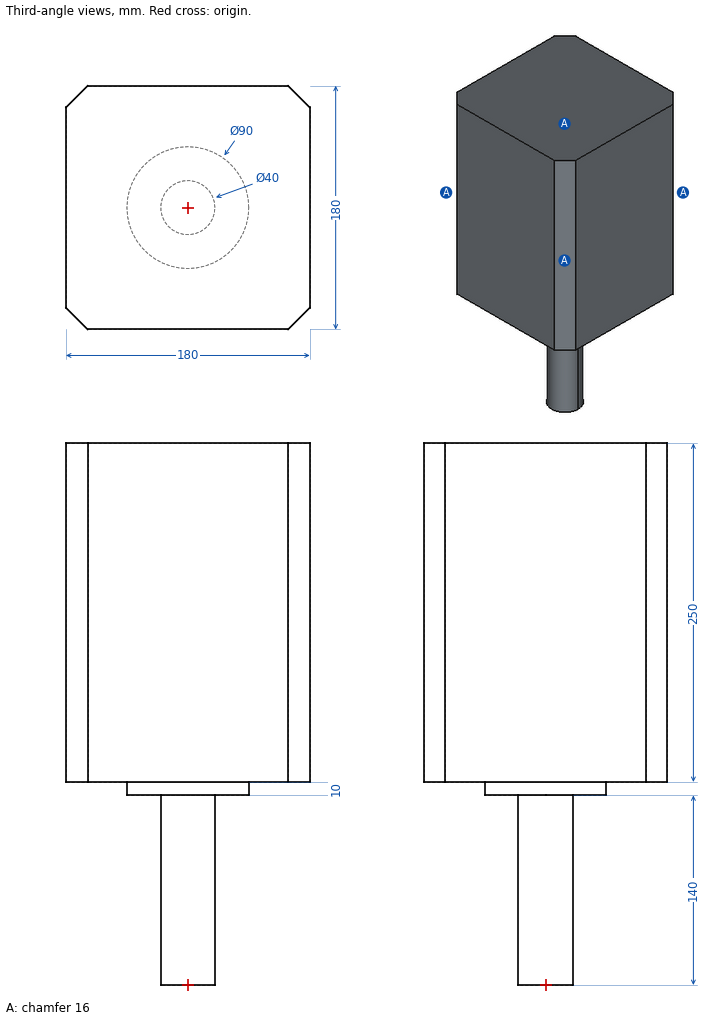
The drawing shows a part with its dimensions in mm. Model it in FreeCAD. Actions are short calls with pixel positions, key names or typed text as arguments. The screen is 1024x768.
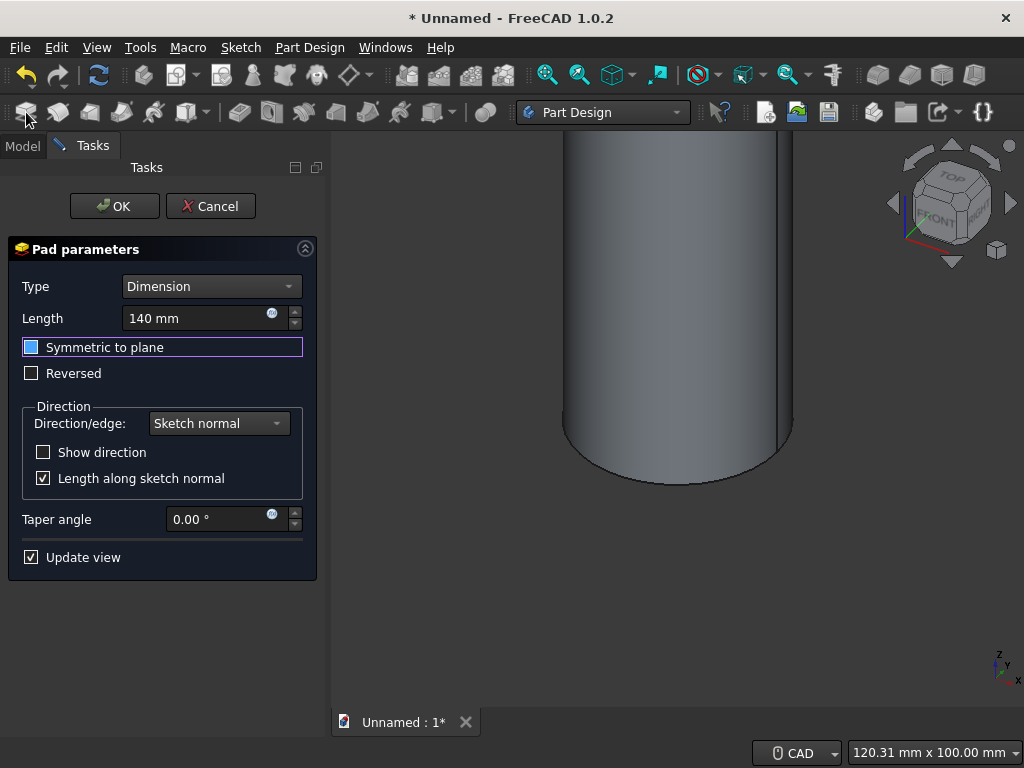
click(115, 206)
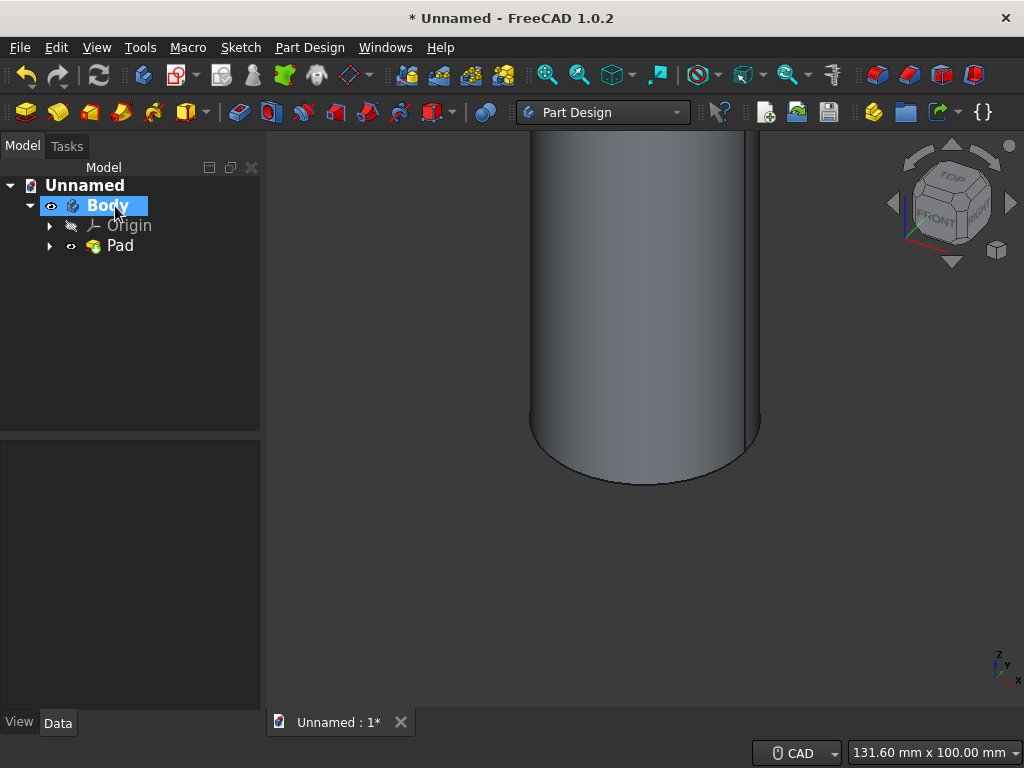
click(548, 76)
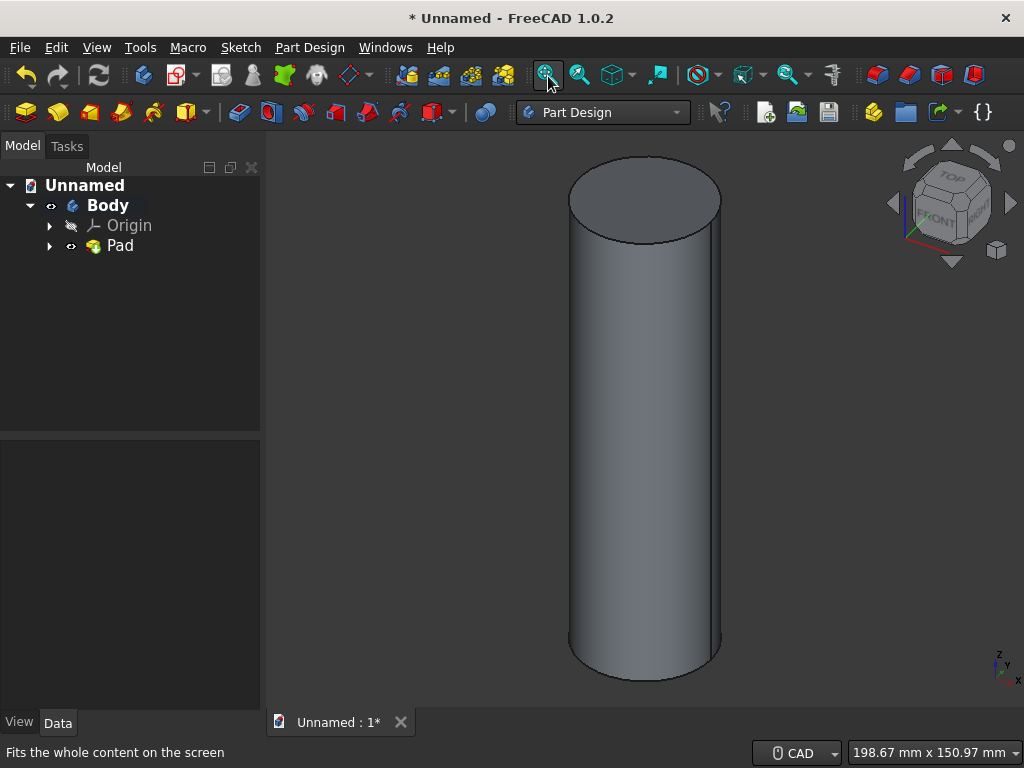
click(645, 199)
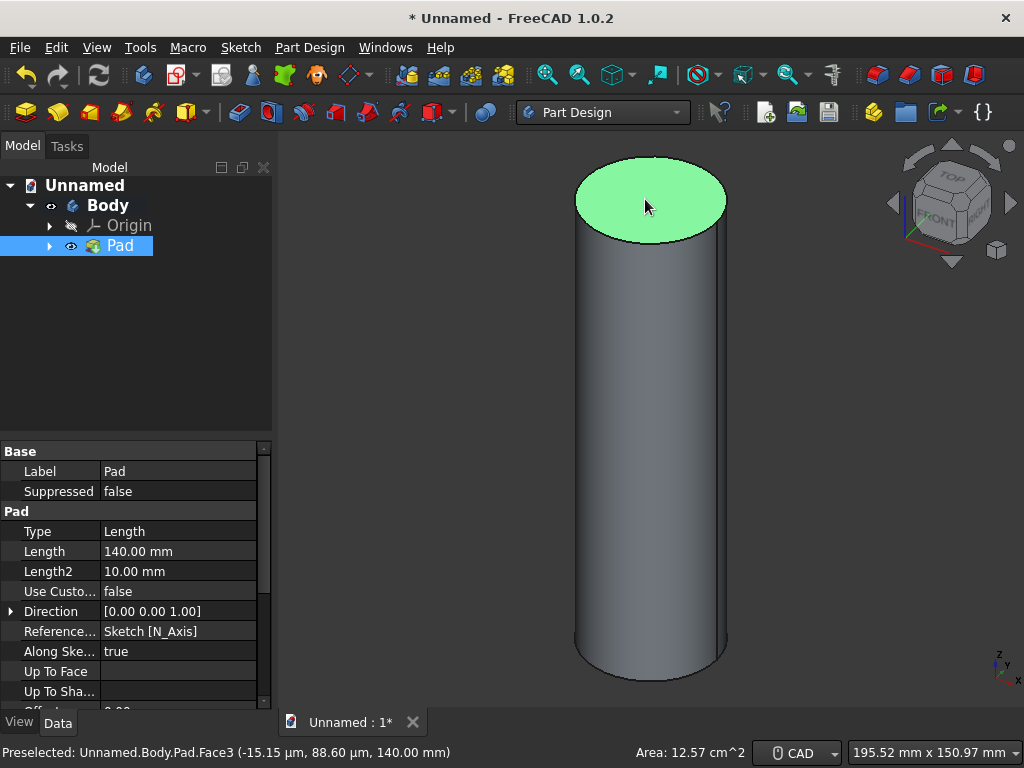
click(176, 76)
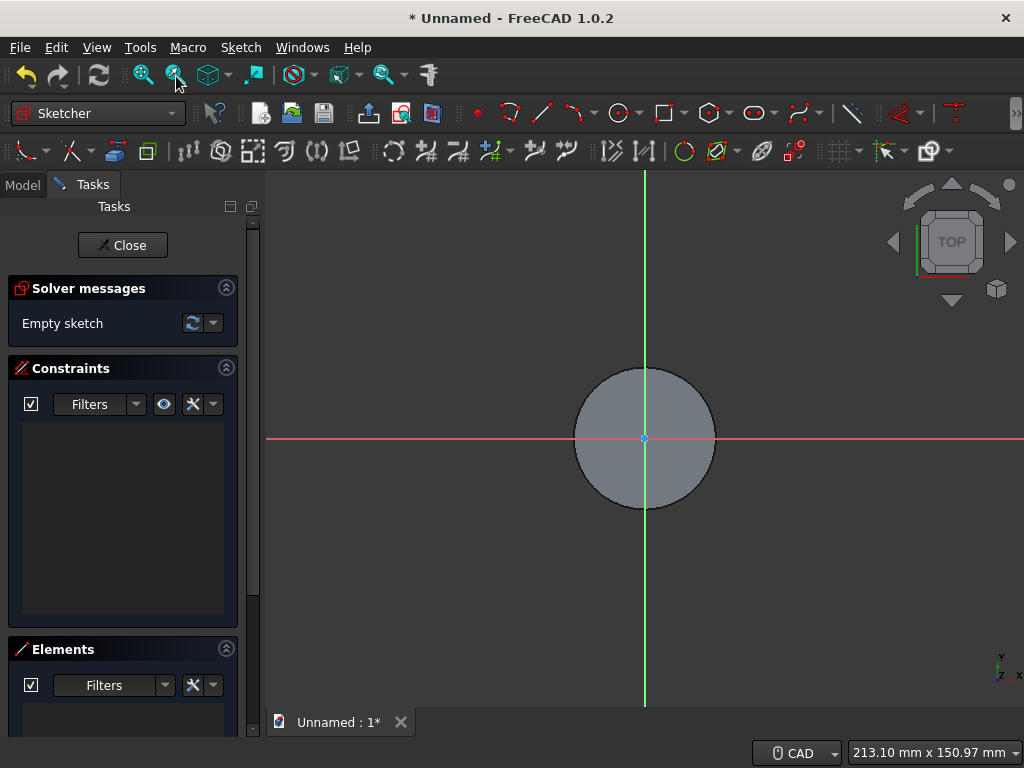
click(620, 114)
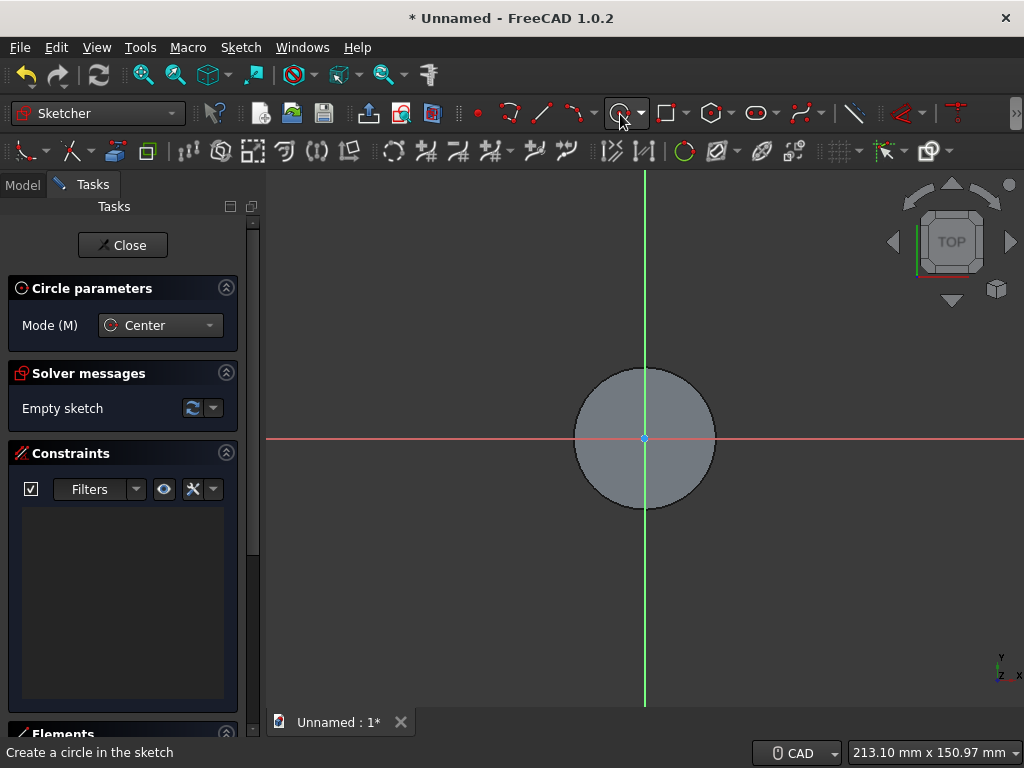
click(645, 438)
click(758, 325)
key(Escape)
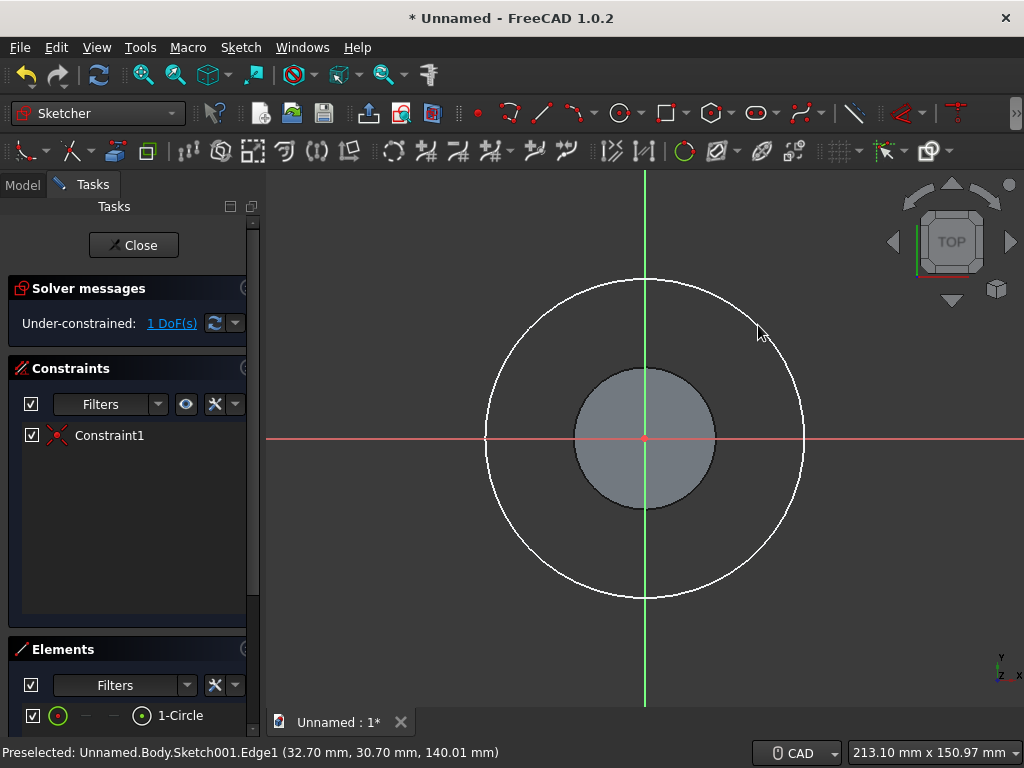
click(902, 114)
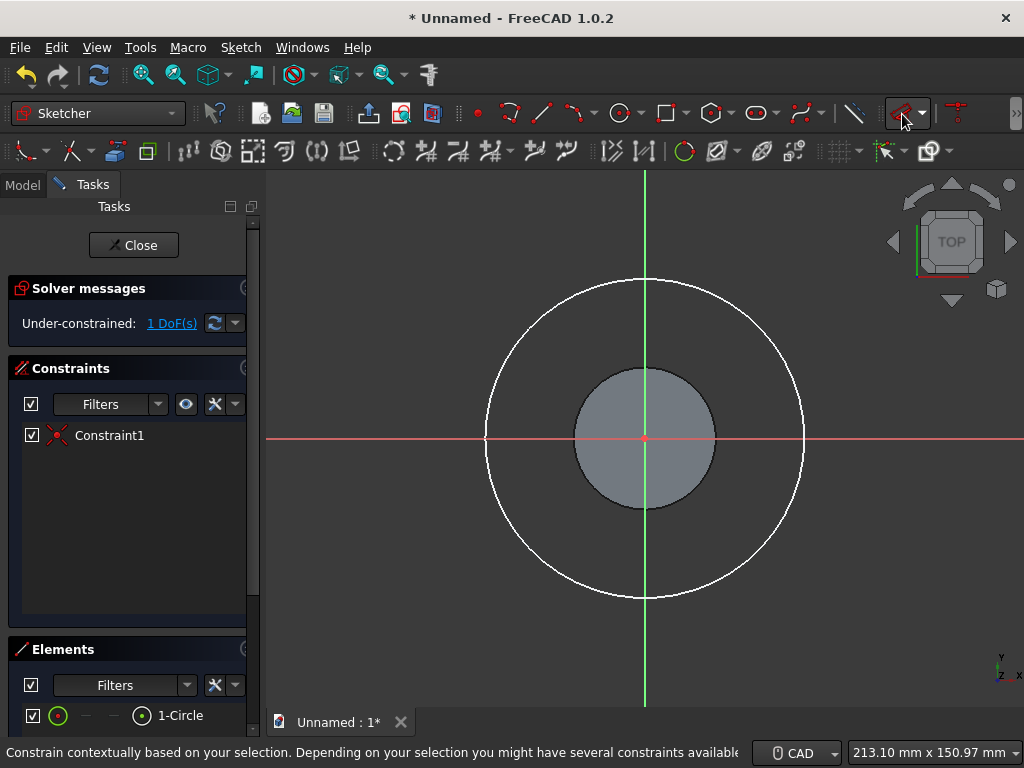
click(757, 325)
click(779, 302)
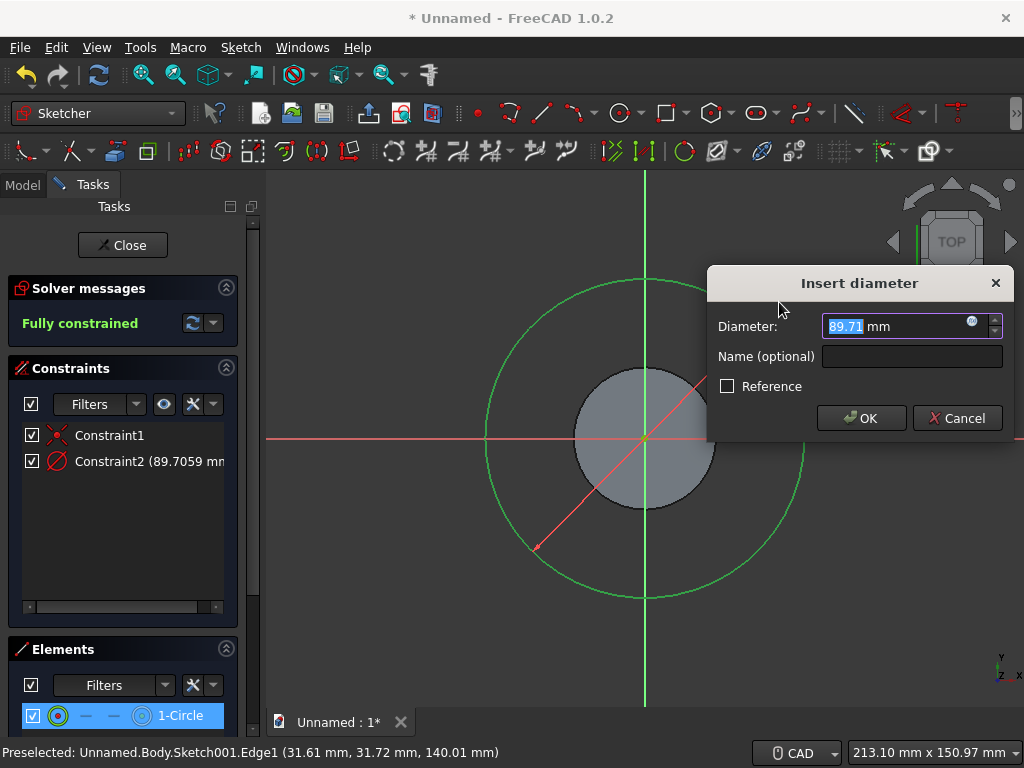
text(90)
key(Return)
key(Escape)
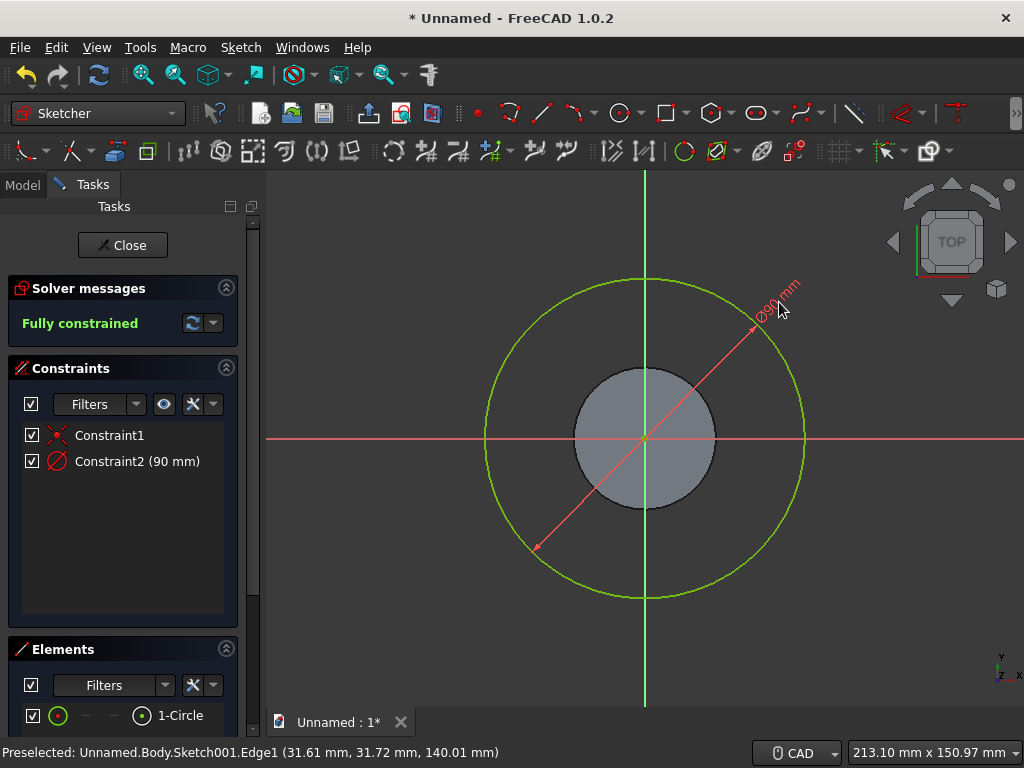
click(123, 245)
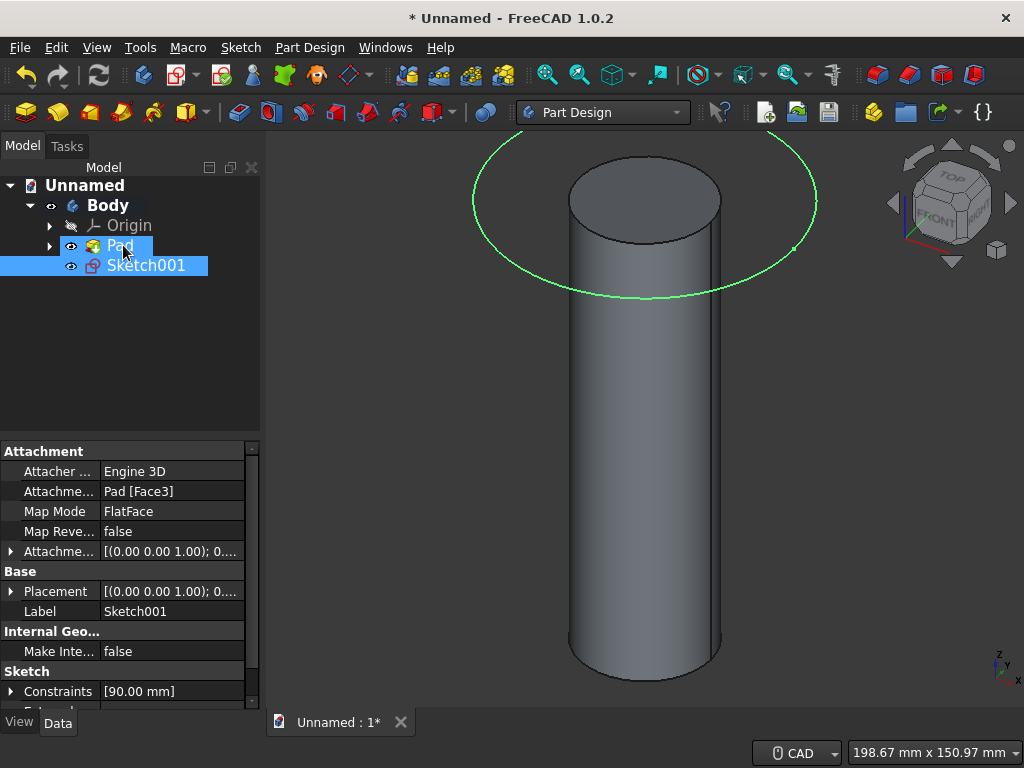
click(26, 112)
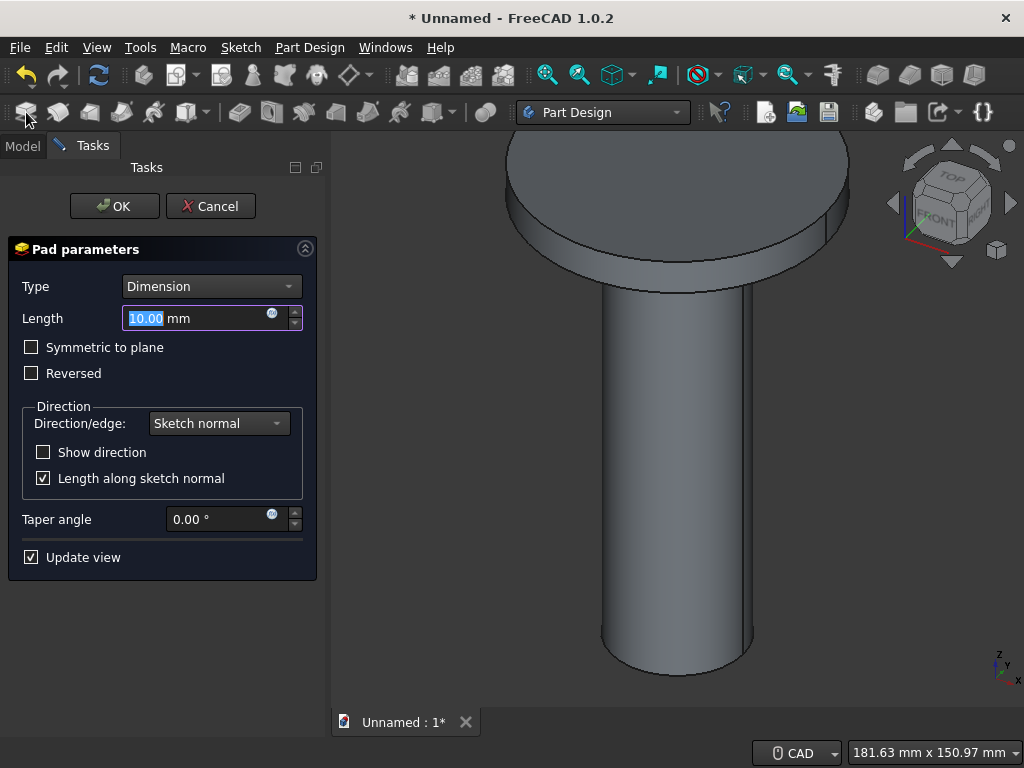
text(10)
key(Tab)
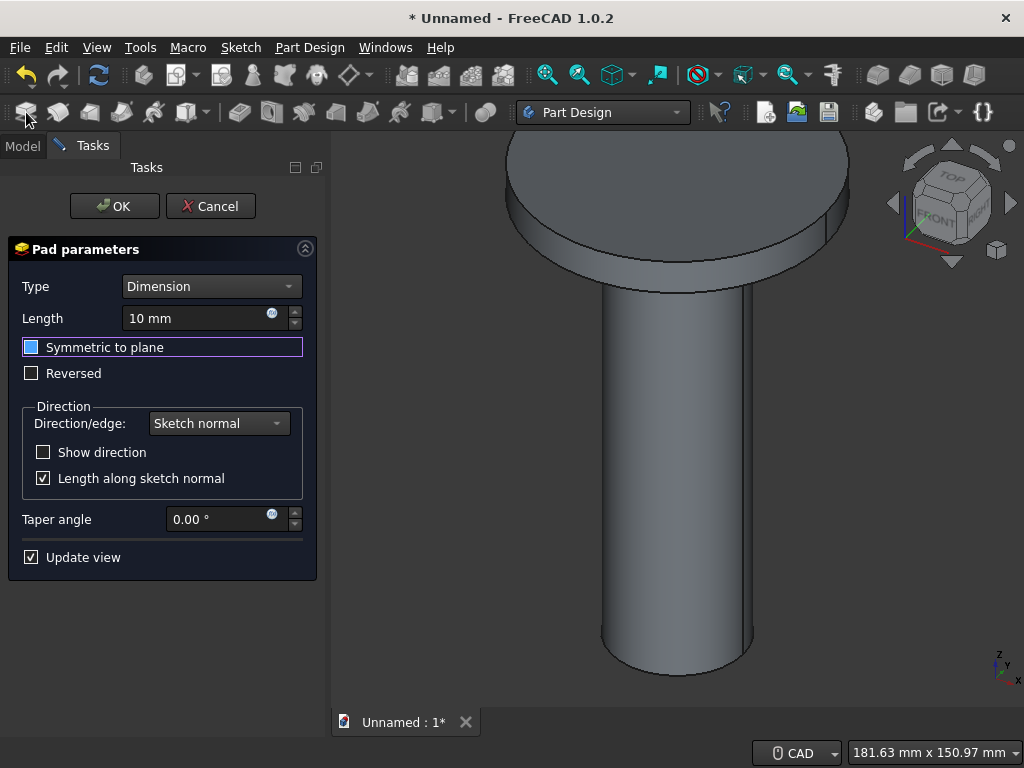
click(115, 206)